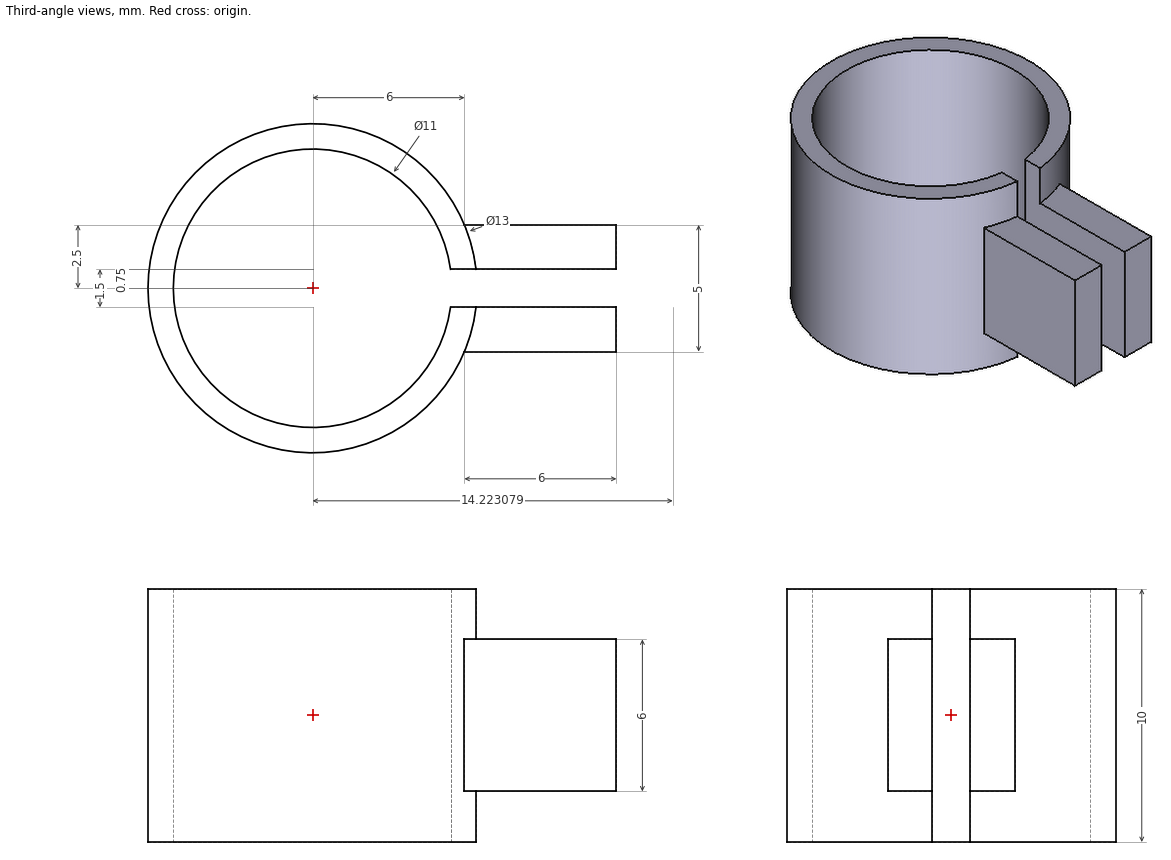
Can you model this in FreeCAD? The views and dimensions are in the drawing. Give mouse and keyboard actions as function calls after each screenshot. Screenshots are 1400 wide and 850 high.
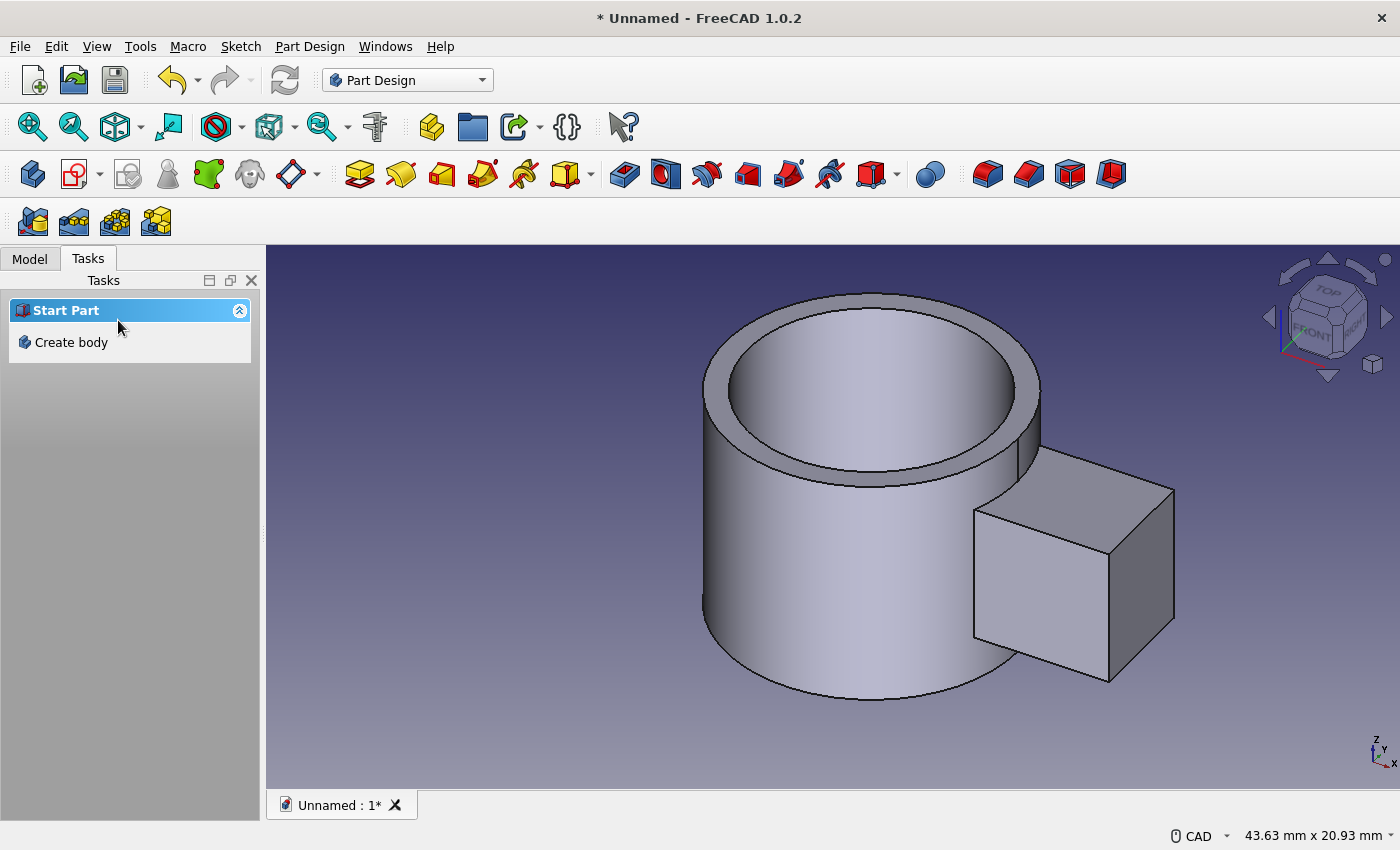
click(1021, 407)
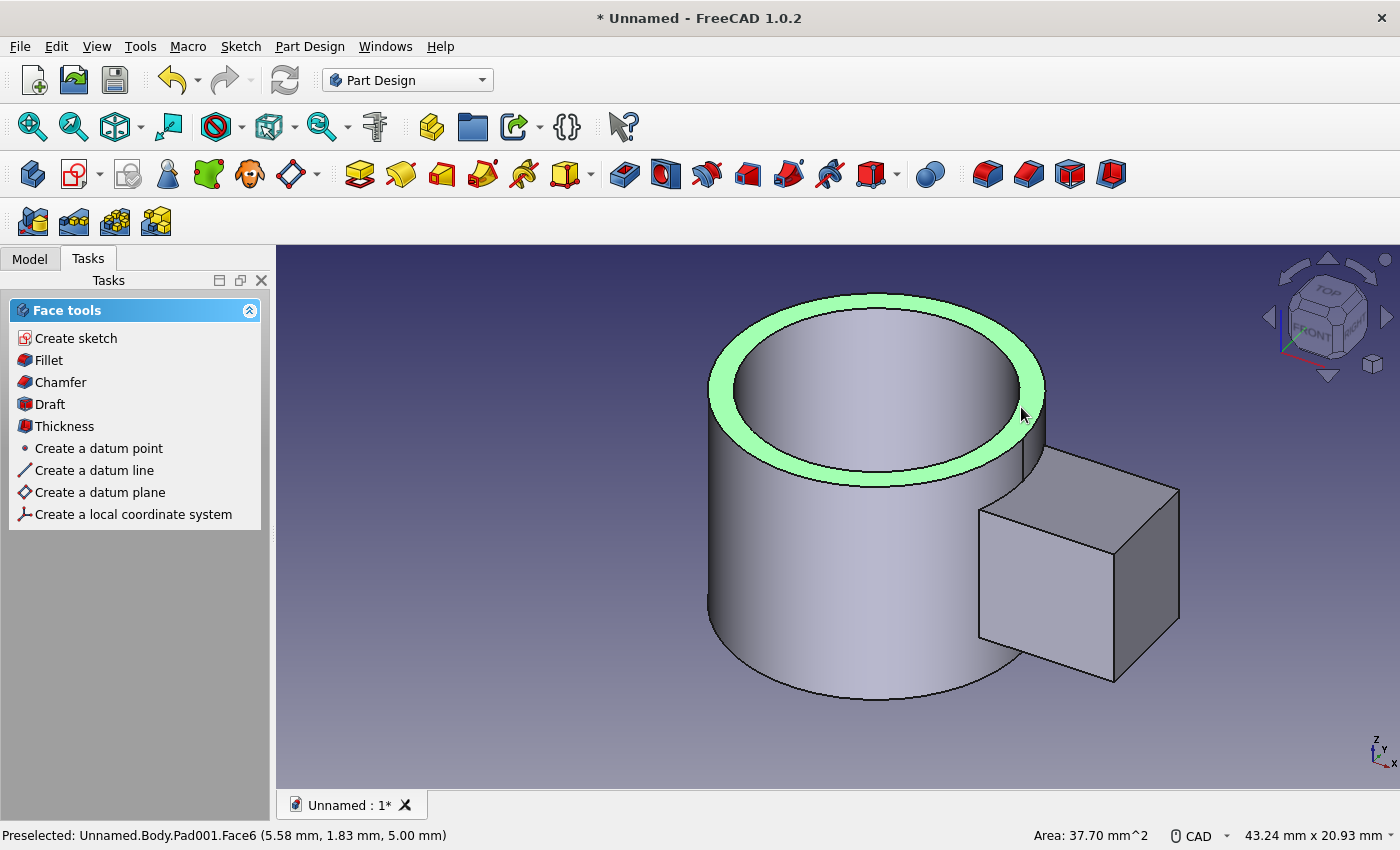
click(74, 174)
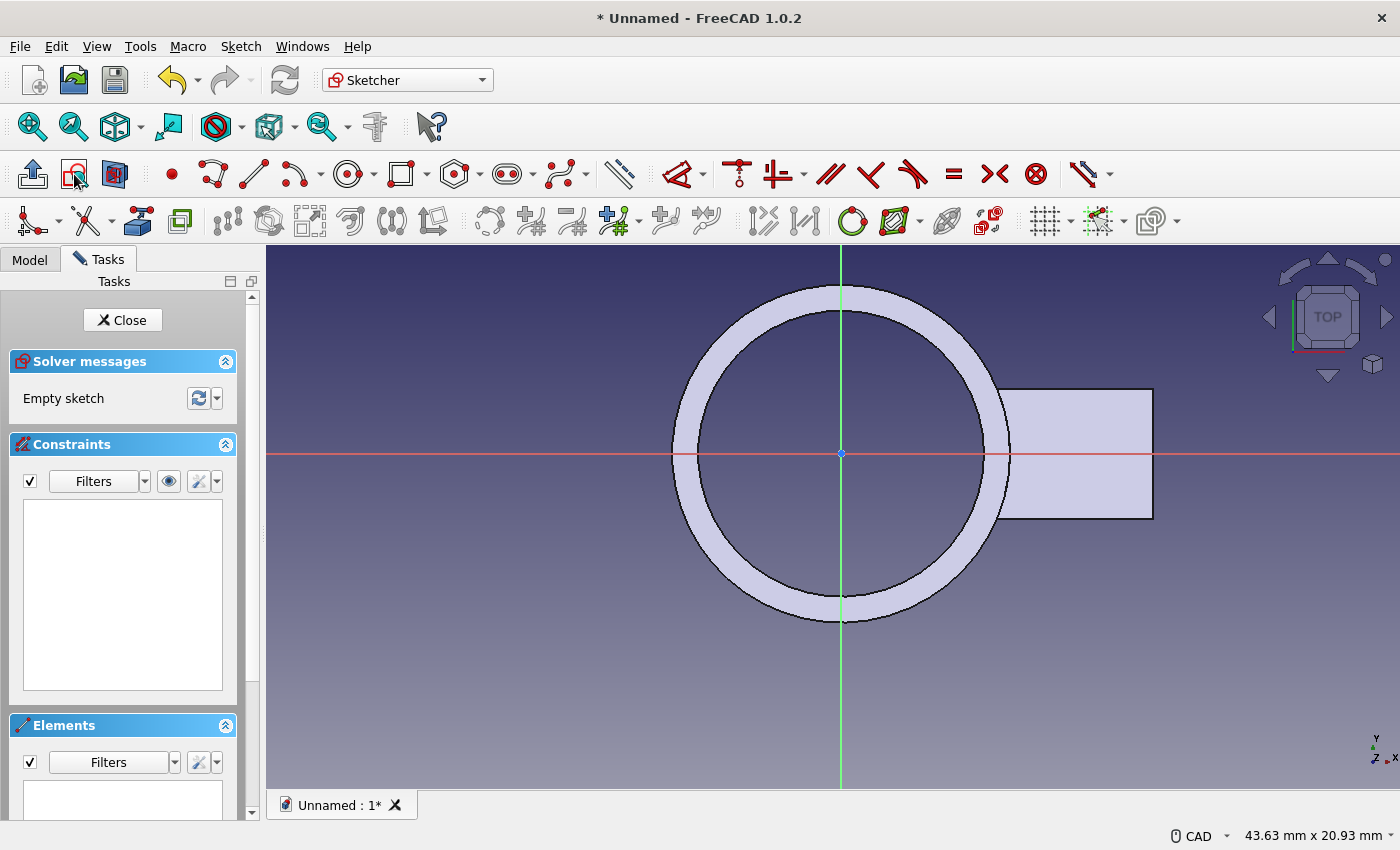
scroll(1235, 377, up, 3)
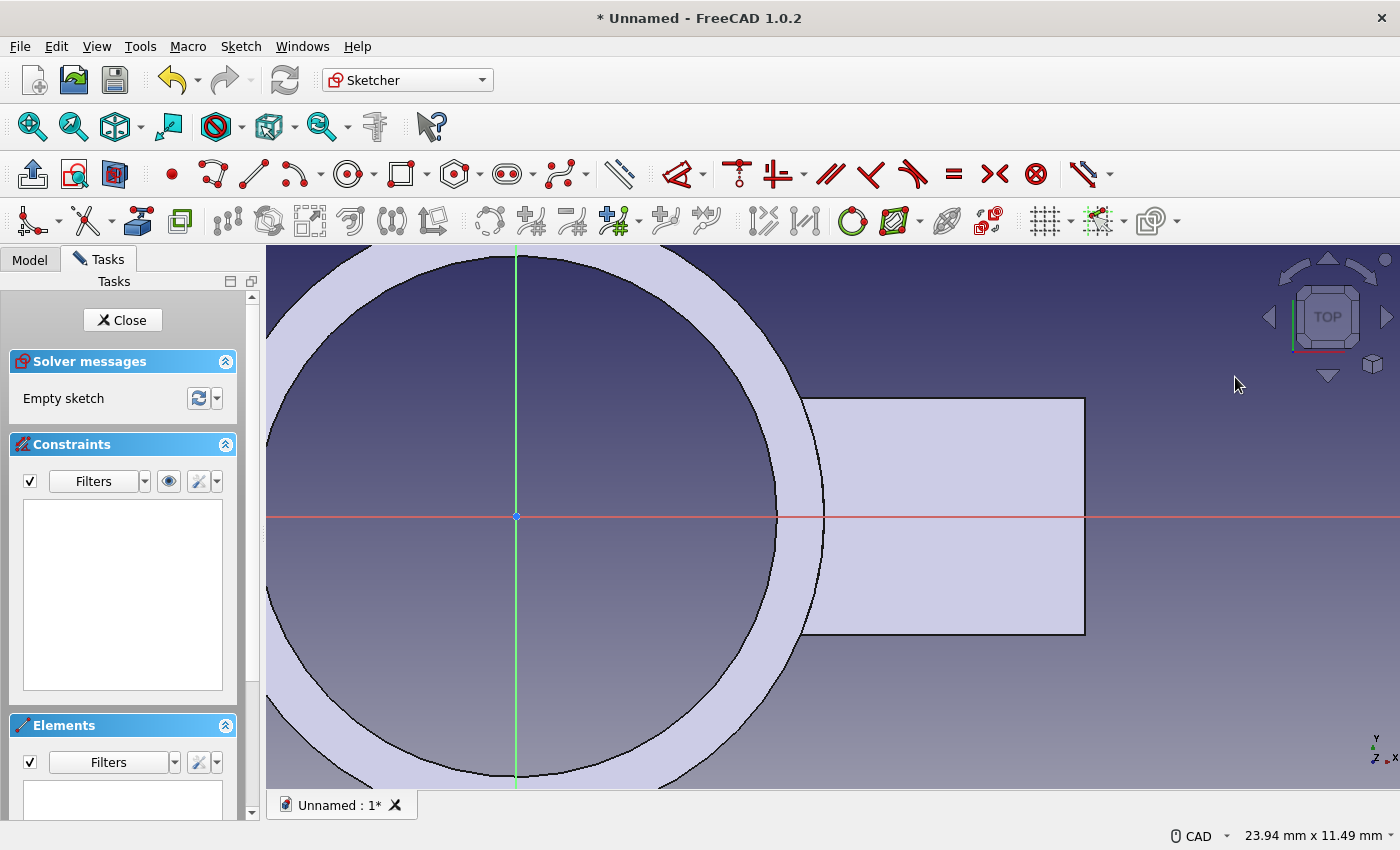
click(400, 174)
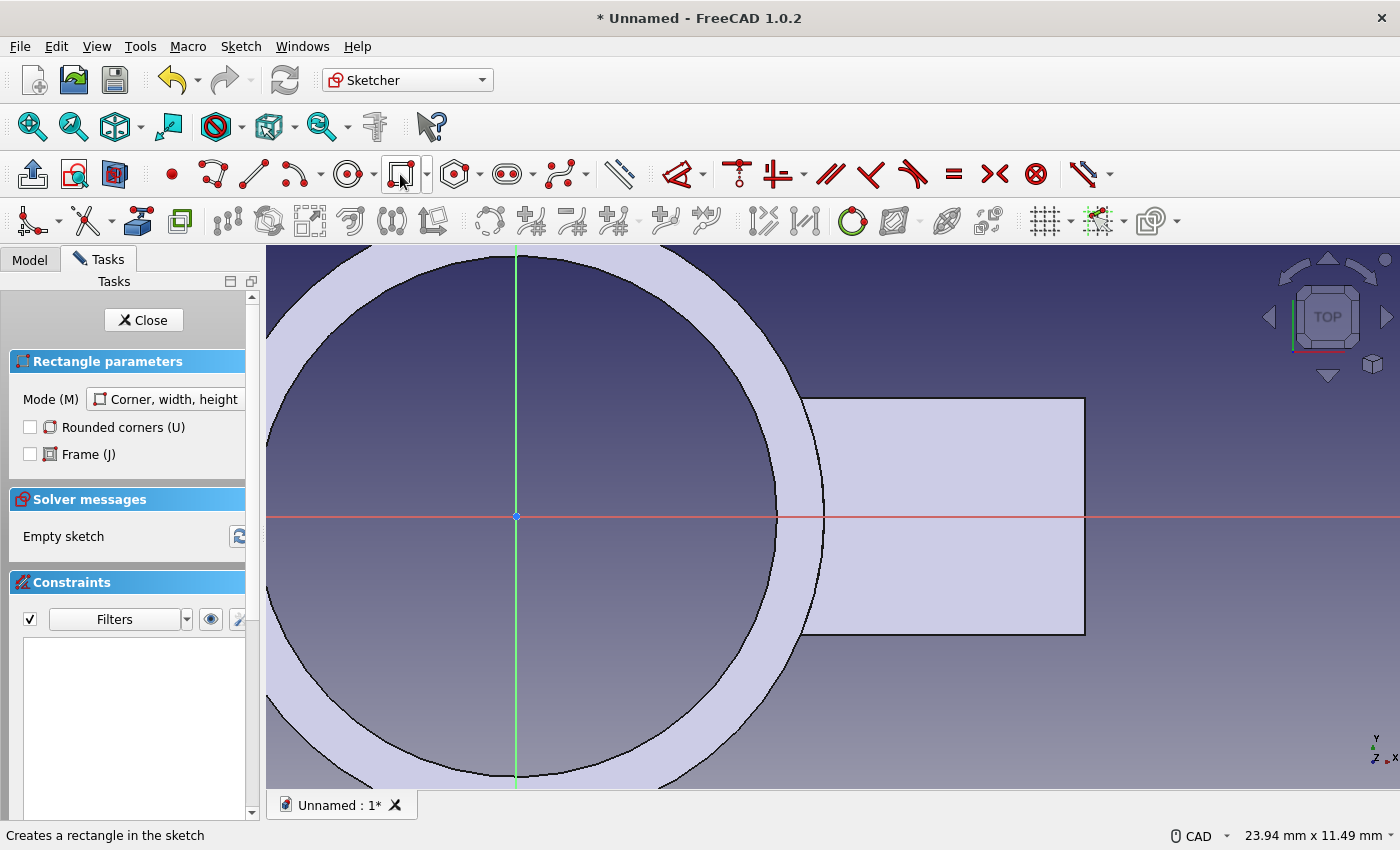
click(516, 481)
click(1190, 552)
key(Escape)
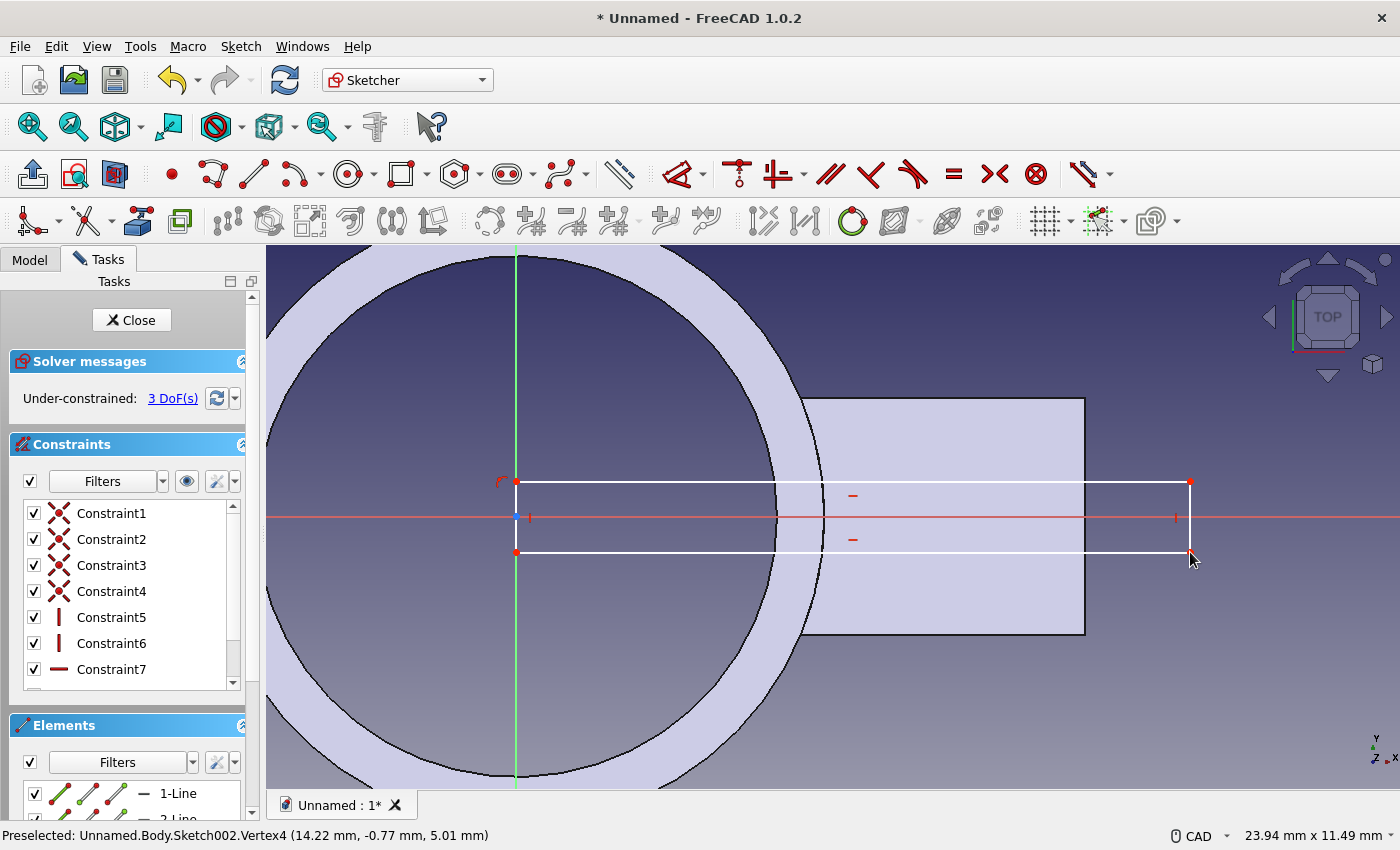
click(676, 174)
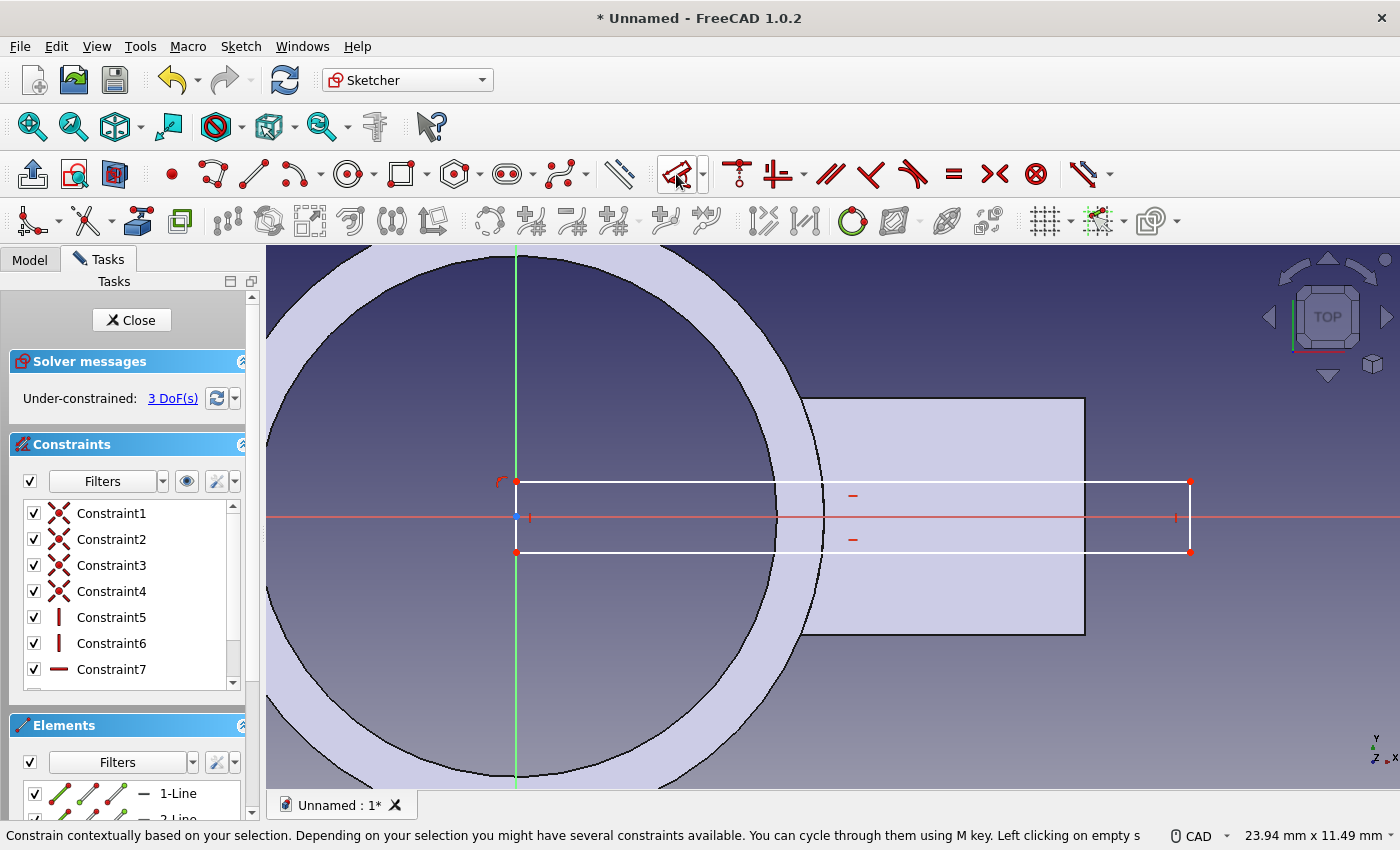
click(516, 503)
click(482, 501)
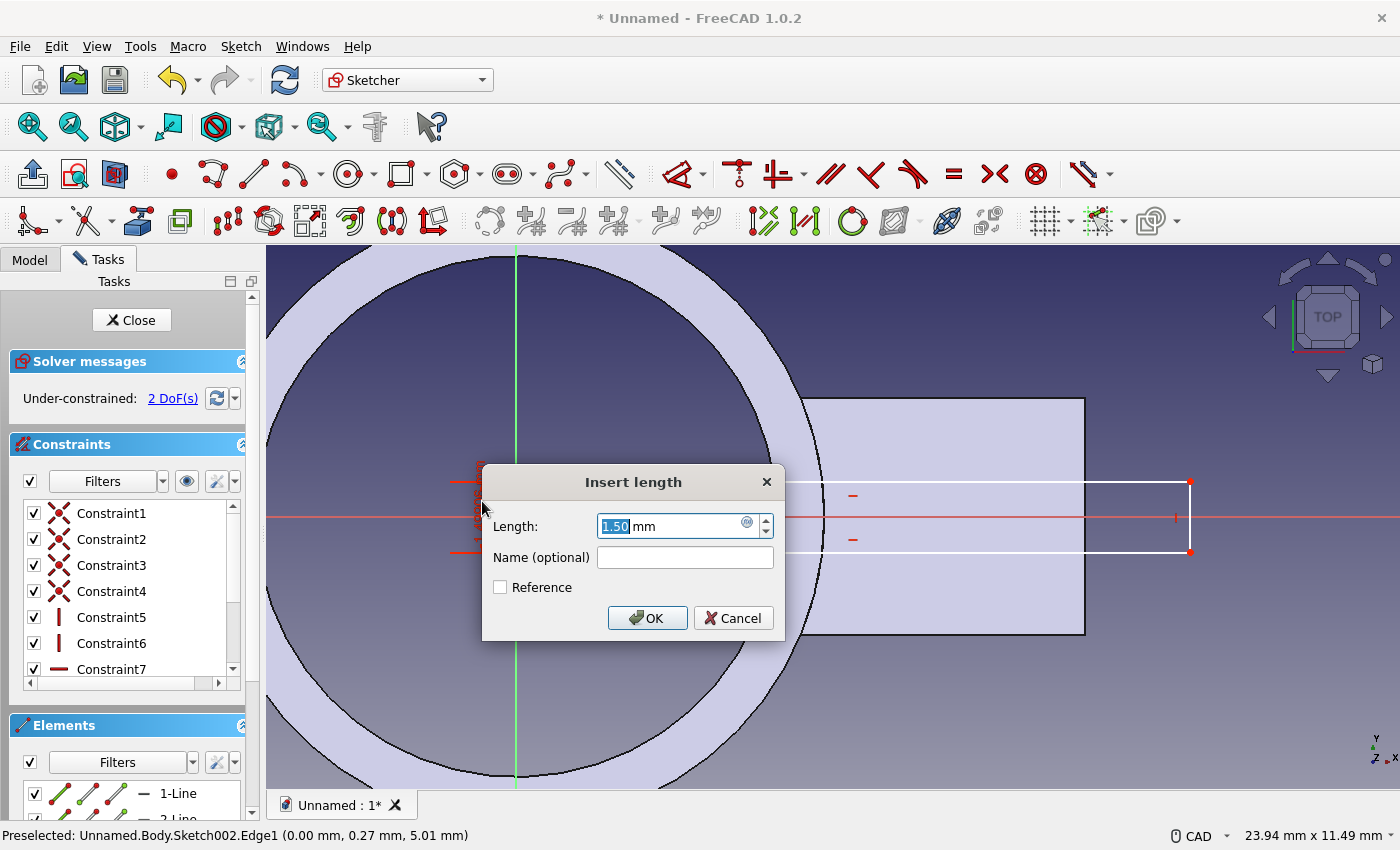
text(1.5)
key(Return)